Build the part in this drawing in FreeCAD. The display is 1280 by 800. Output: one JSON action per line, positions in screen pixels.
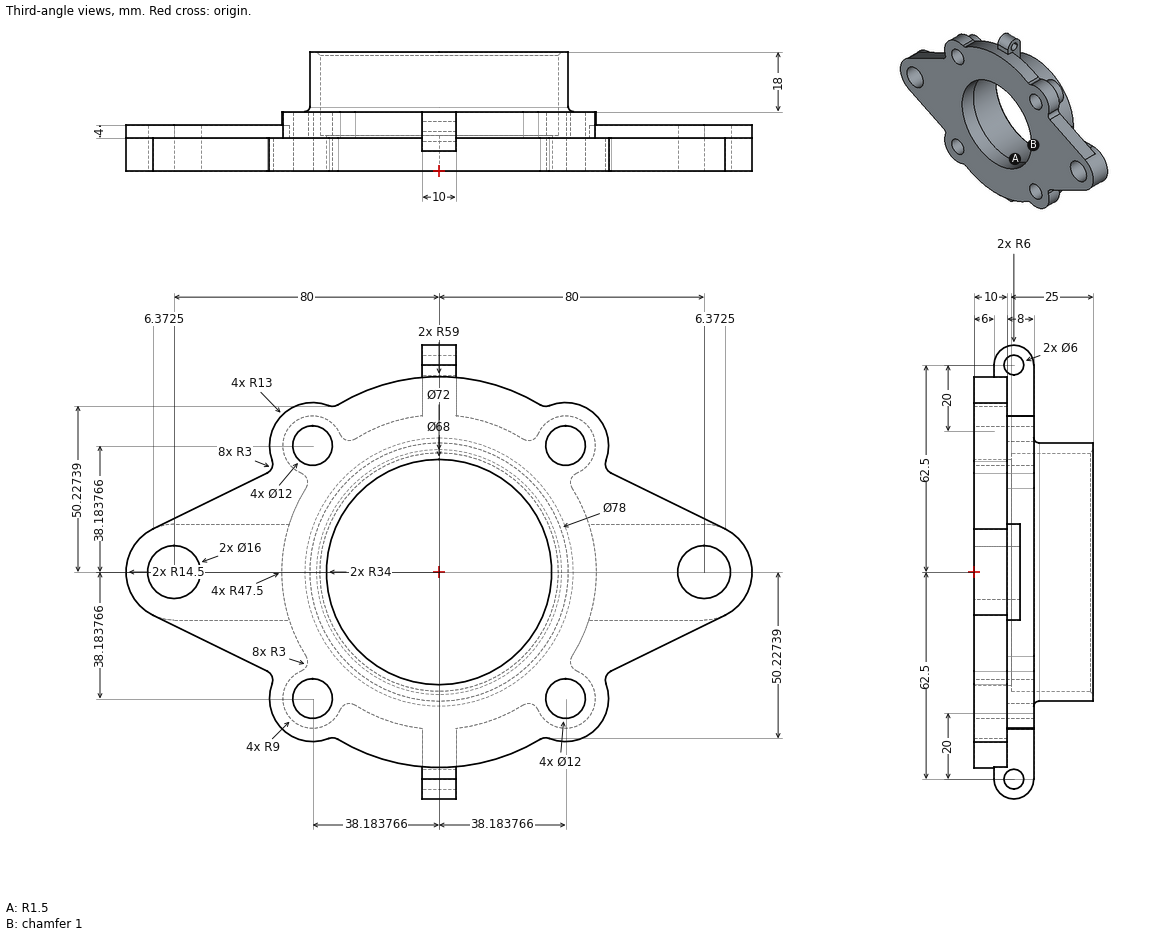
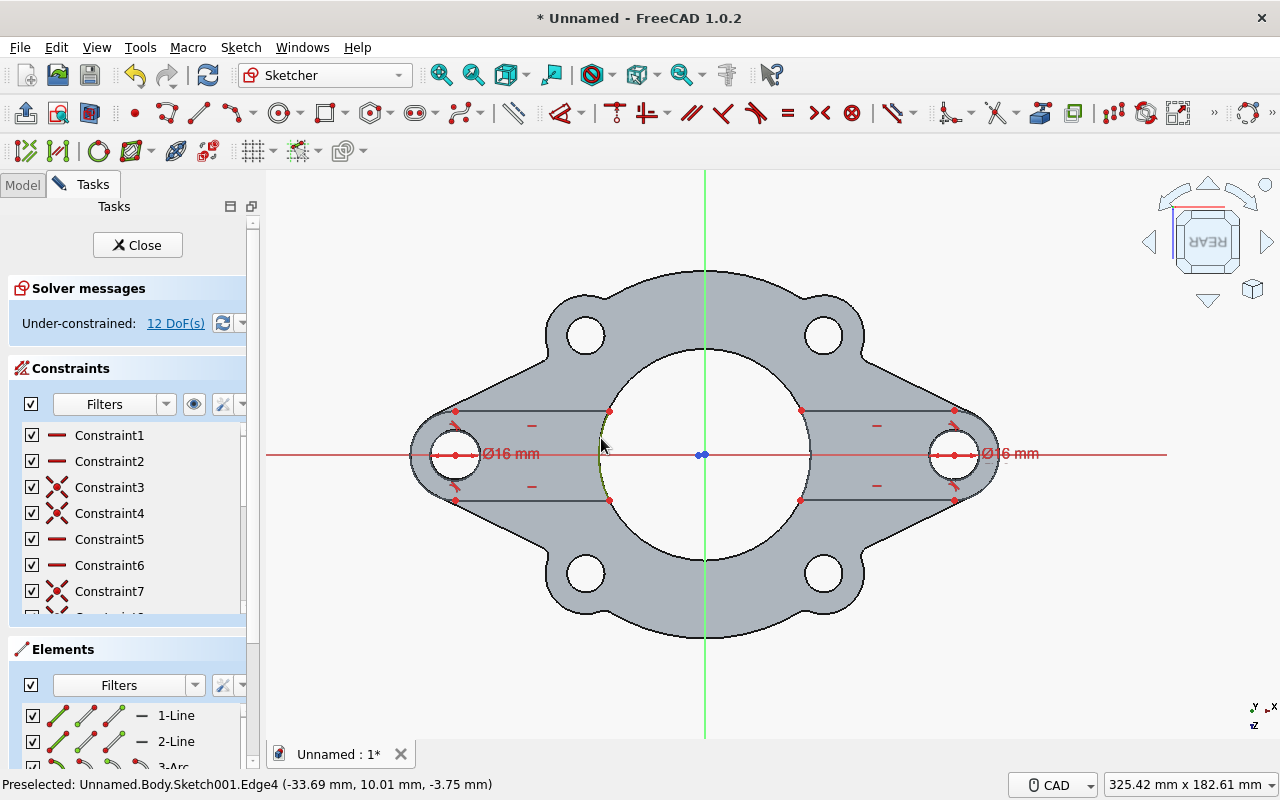
{"action": "left_click", "coordinate": [809, 474]}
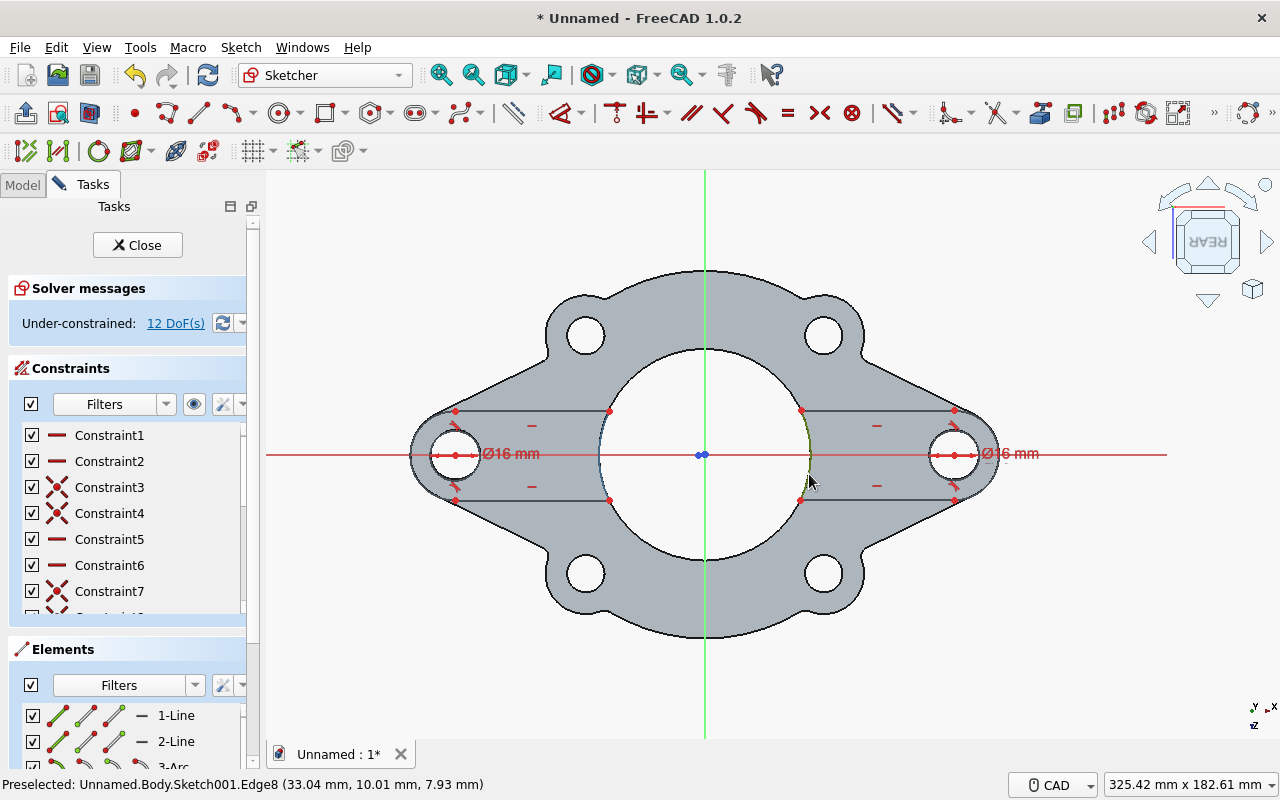
{"action": "left_click", "coordinate": [616, 114]}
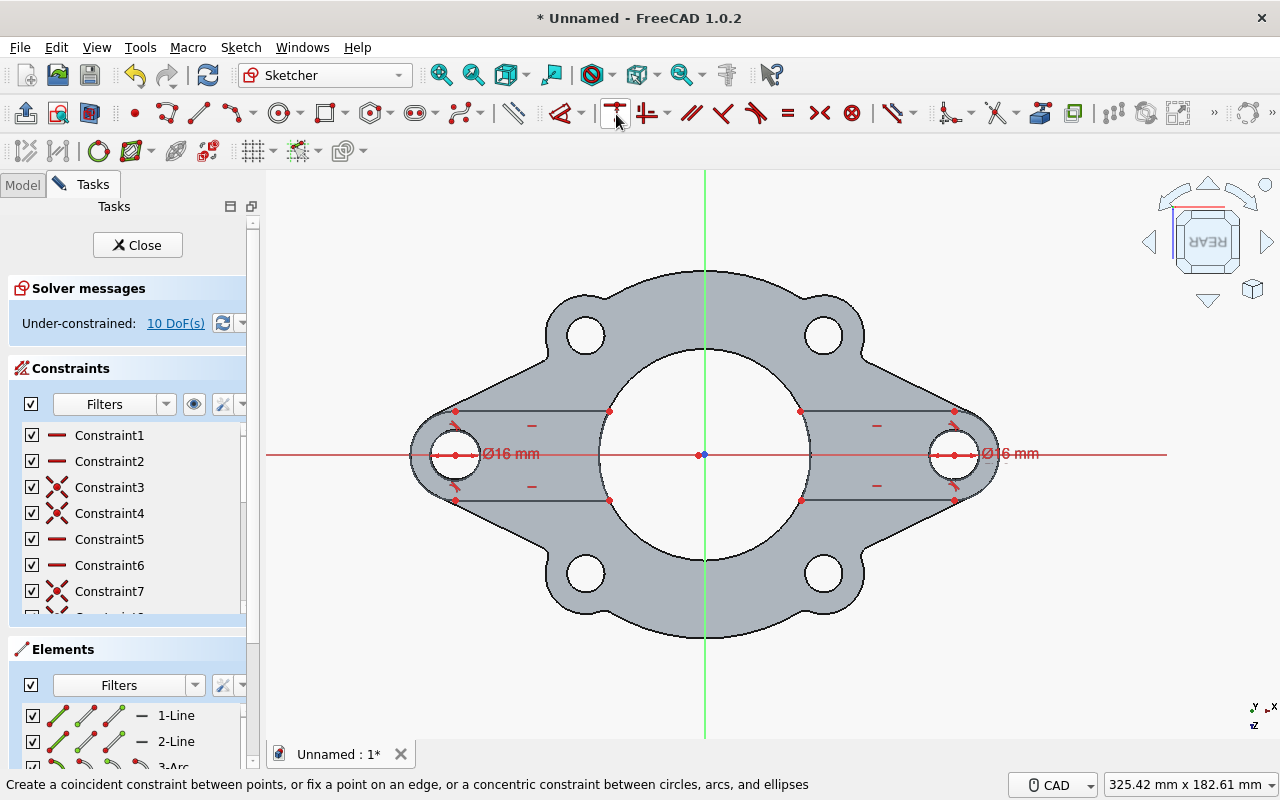
{"action": "scroll", "coordinate": [702, 455], "scroll_direction": "up", "scroll_amount": 3}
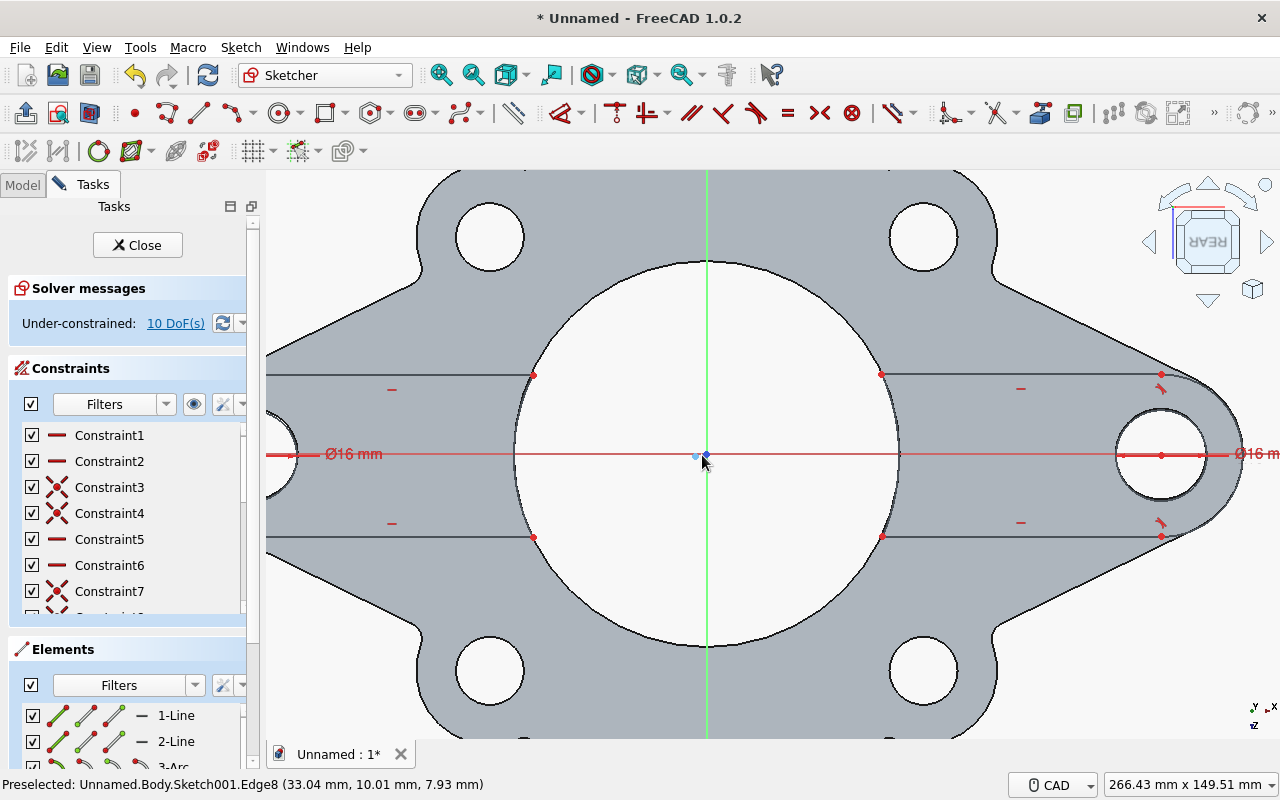
{"action": "left_click_drag", "start_coordinate": [685, 444], "coordinate": [717, 466]}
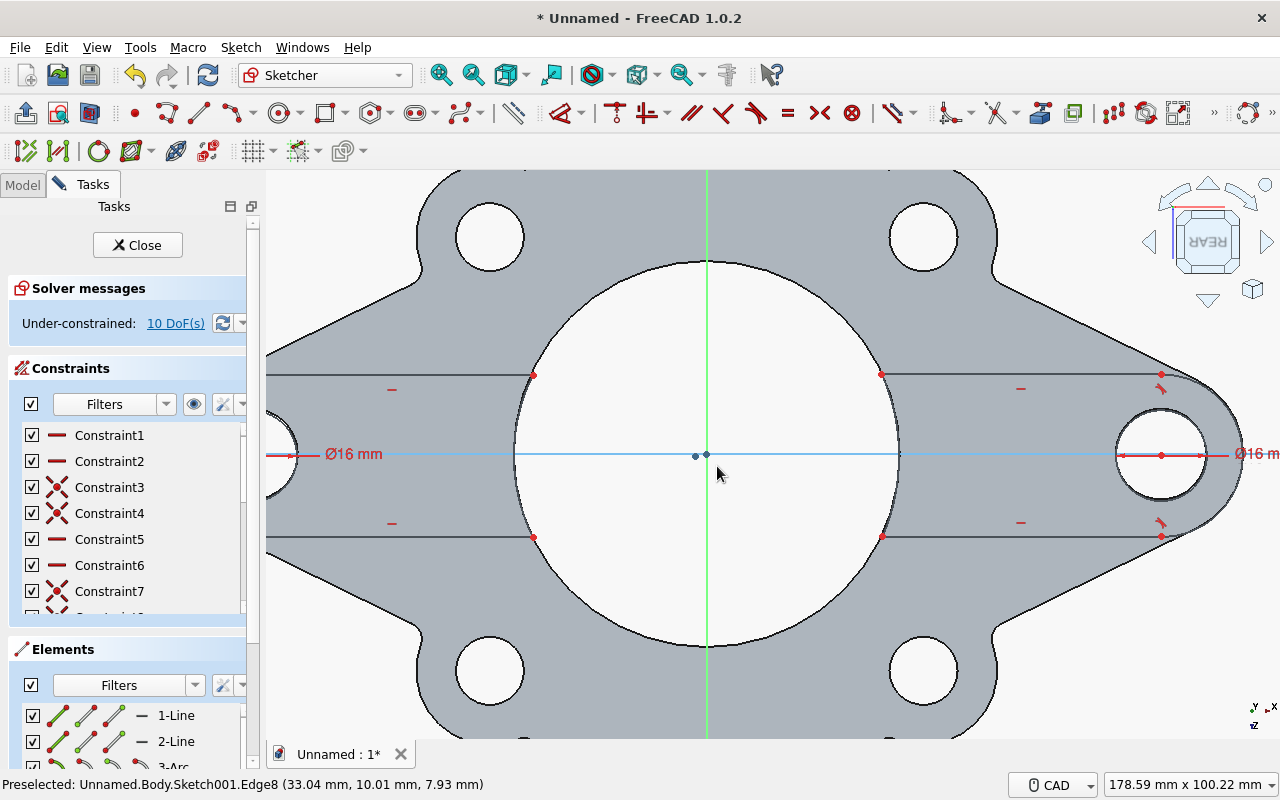
{"action": "left_click", "coordinate": [616, 114]}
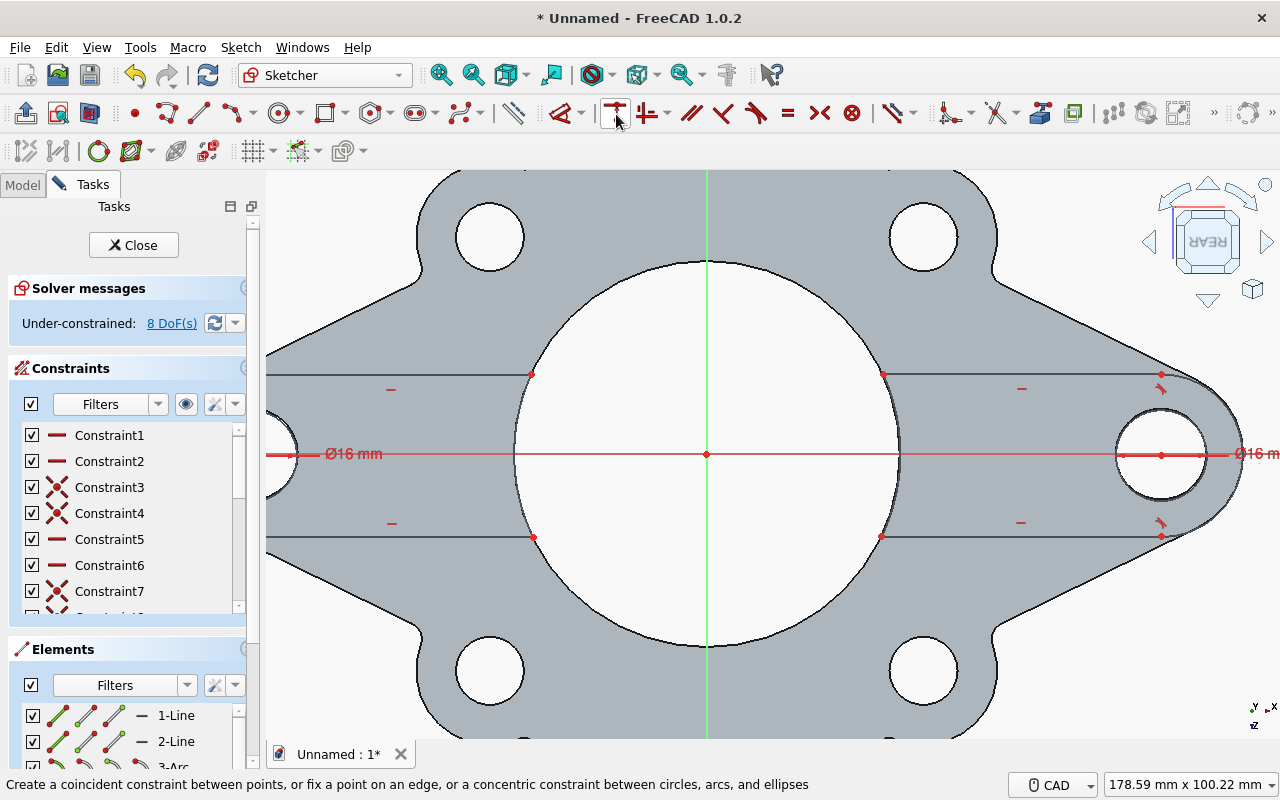
{"action": "scroll", "coordinate": [702, 455], "scroll_direction": "down", "scroll_amount": 3}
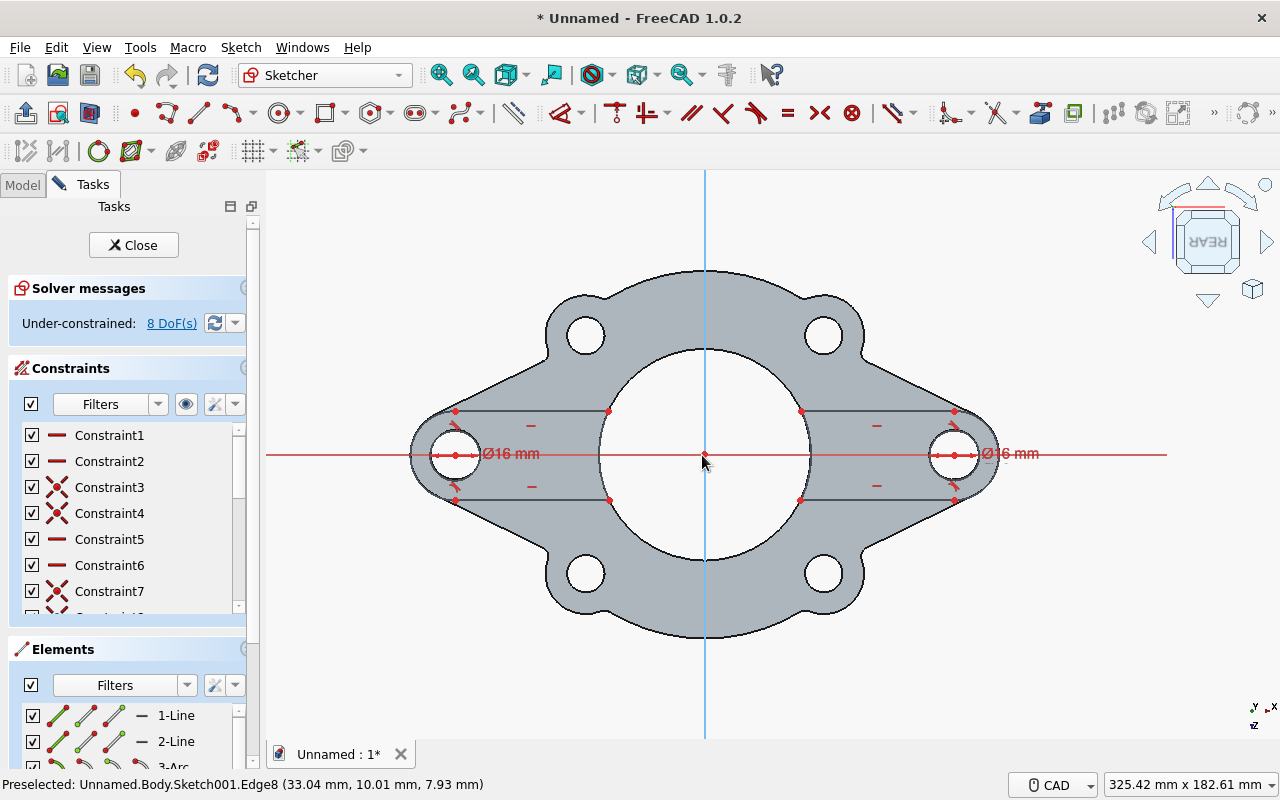
{"action": "left_click", "coordinate": [419, 430]}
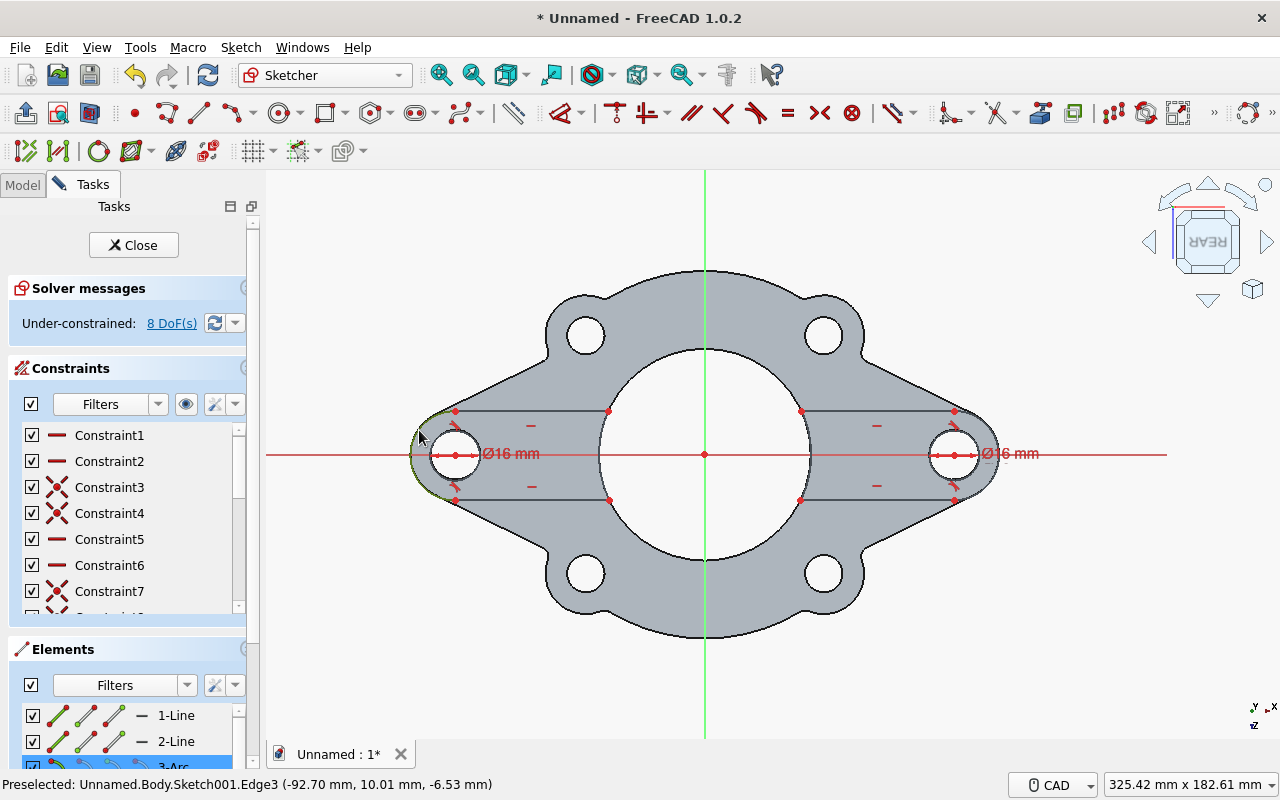
{"action": "left_click", "coordinate": [990, 482]}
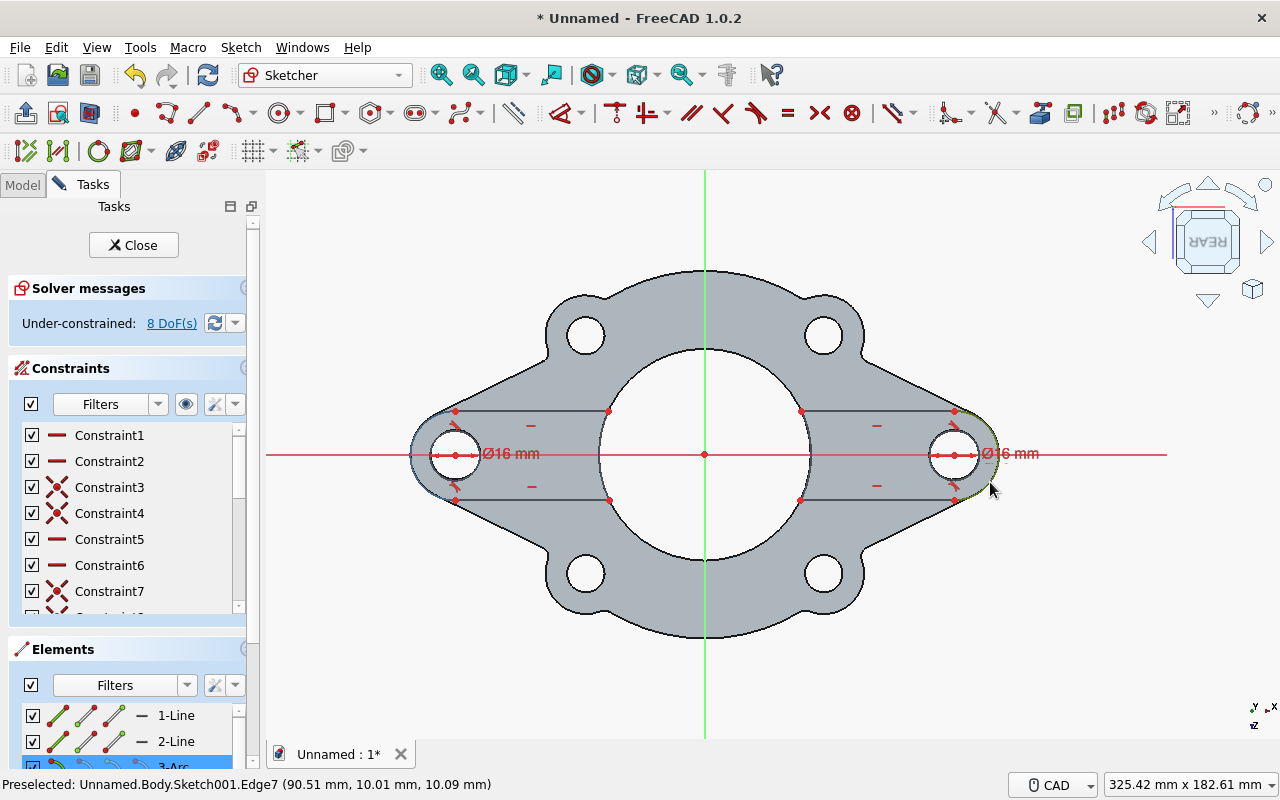
{"action": "left_click", "coordinate": [788, 114]}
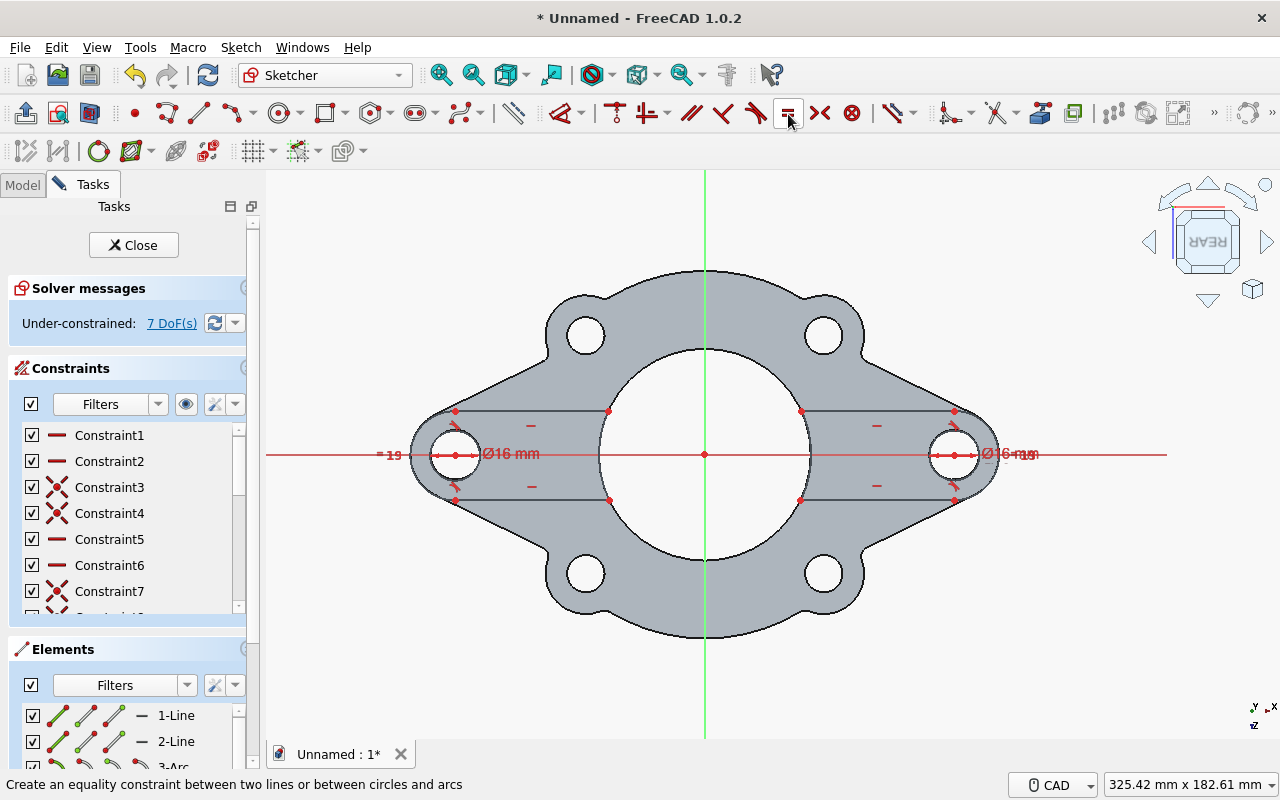
{"action": "left_click", "coordinate": [601, 438]}